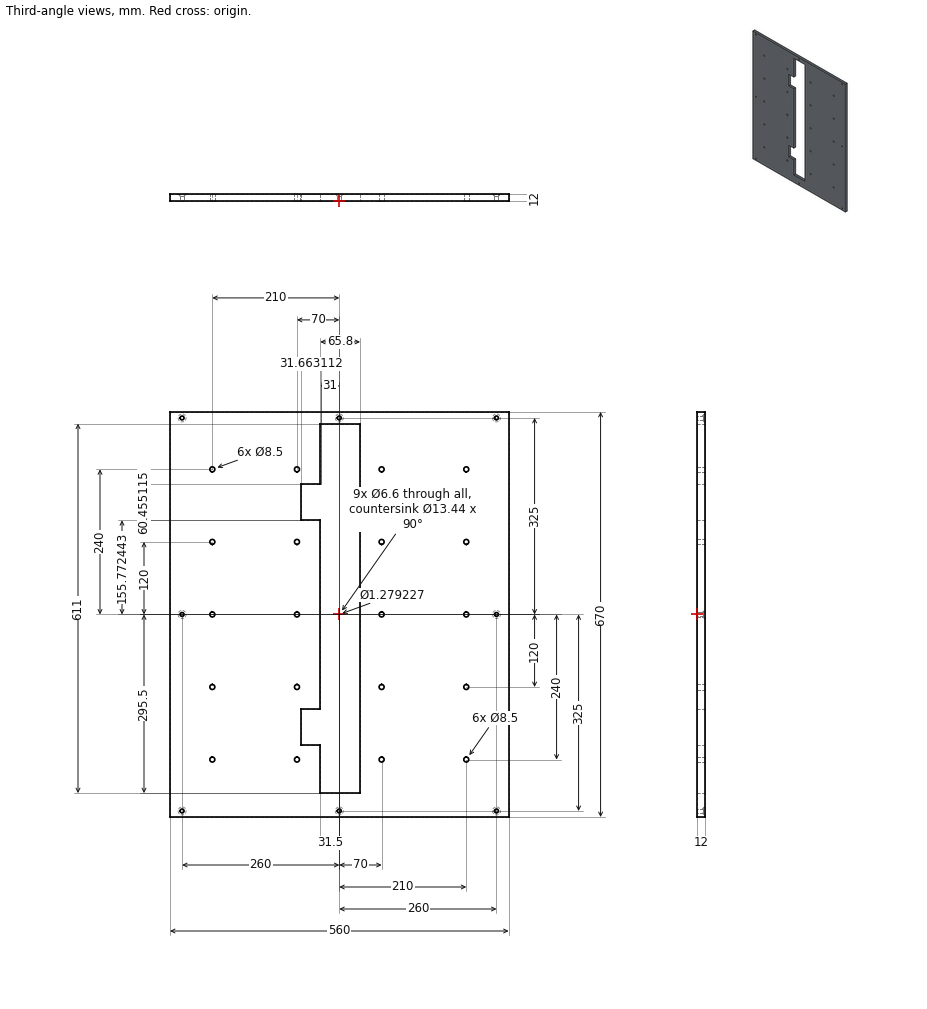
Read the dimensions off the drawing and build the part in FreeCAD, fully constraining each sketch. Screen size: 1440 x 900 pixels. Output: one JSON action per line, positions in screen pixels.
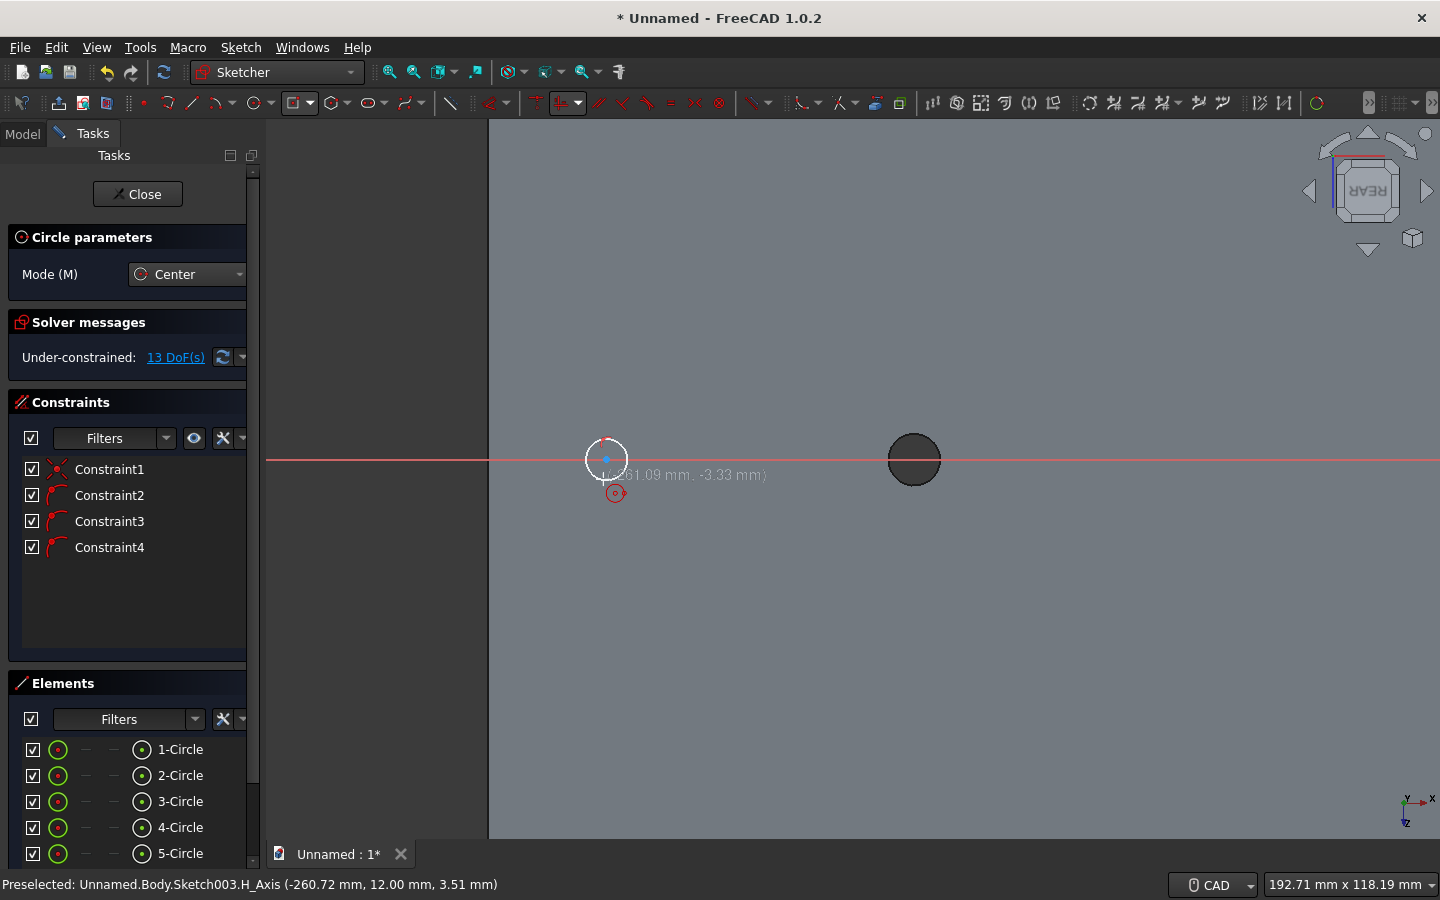
{"action": "scroll", "coordinate": [609, 481], "scroll_direction": "down", "scroll_amount": 11}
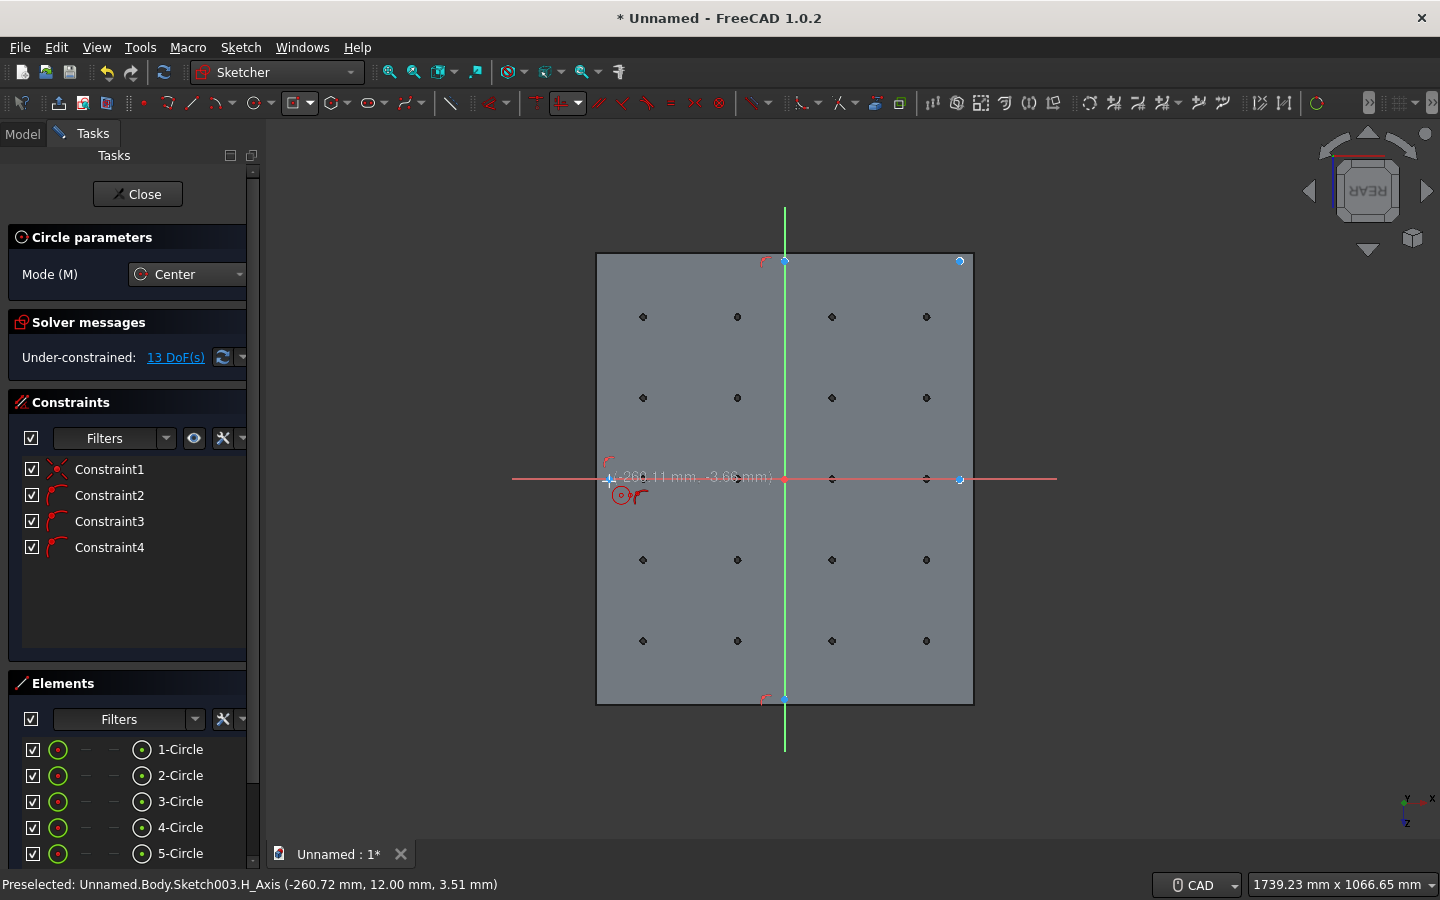
{"action": "scroll", "coordinate": [609, 260], "scroll_direction": "up", "scroll_amount": 12}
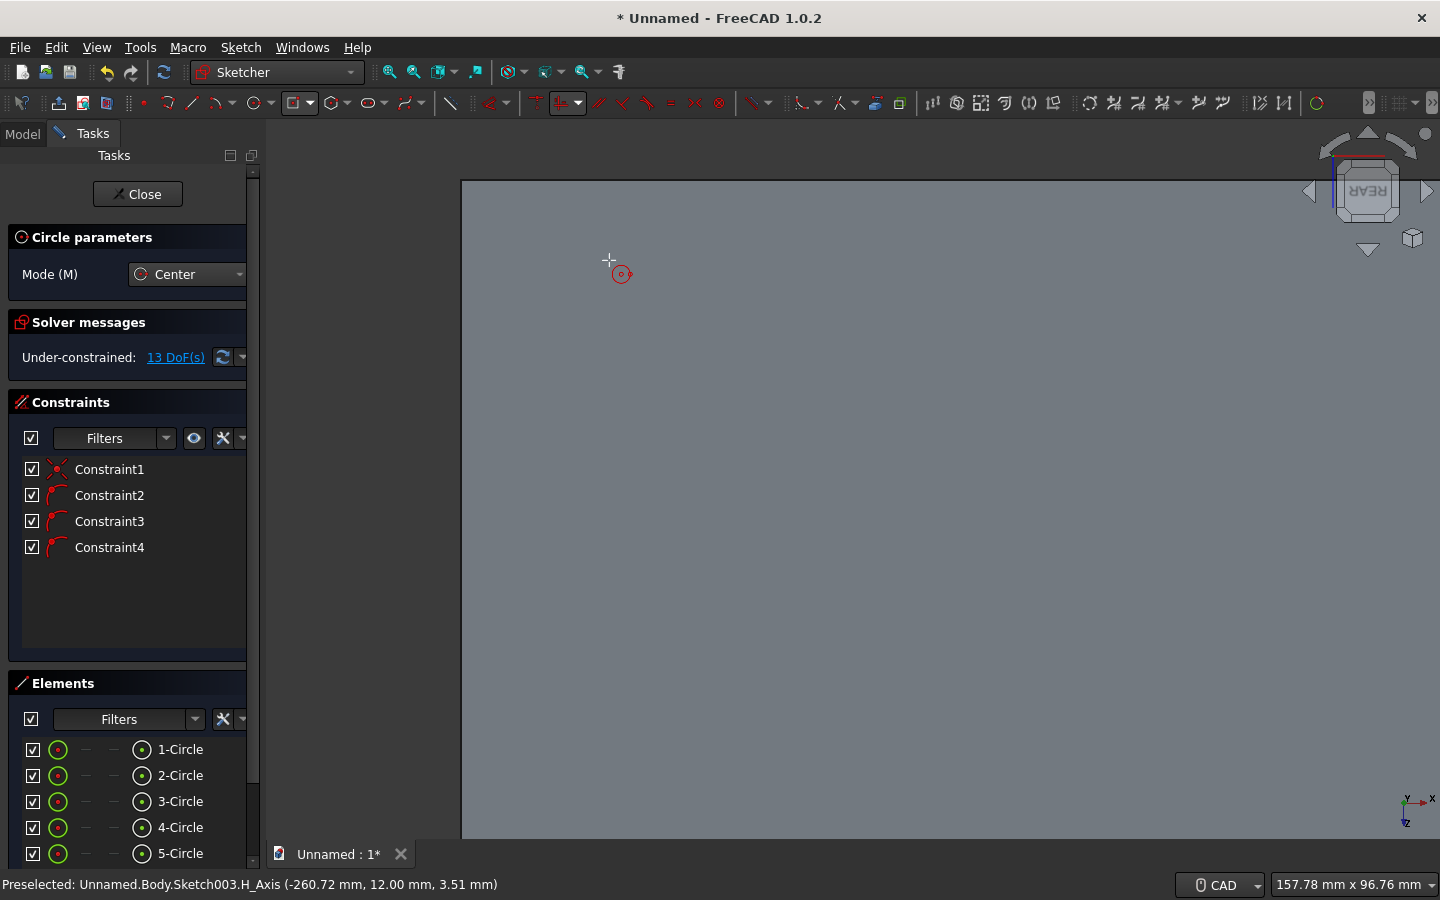
{"action": "scroll", "coordinate": [609, 260], "scroll_direction": "down", "scroll_amount": 12}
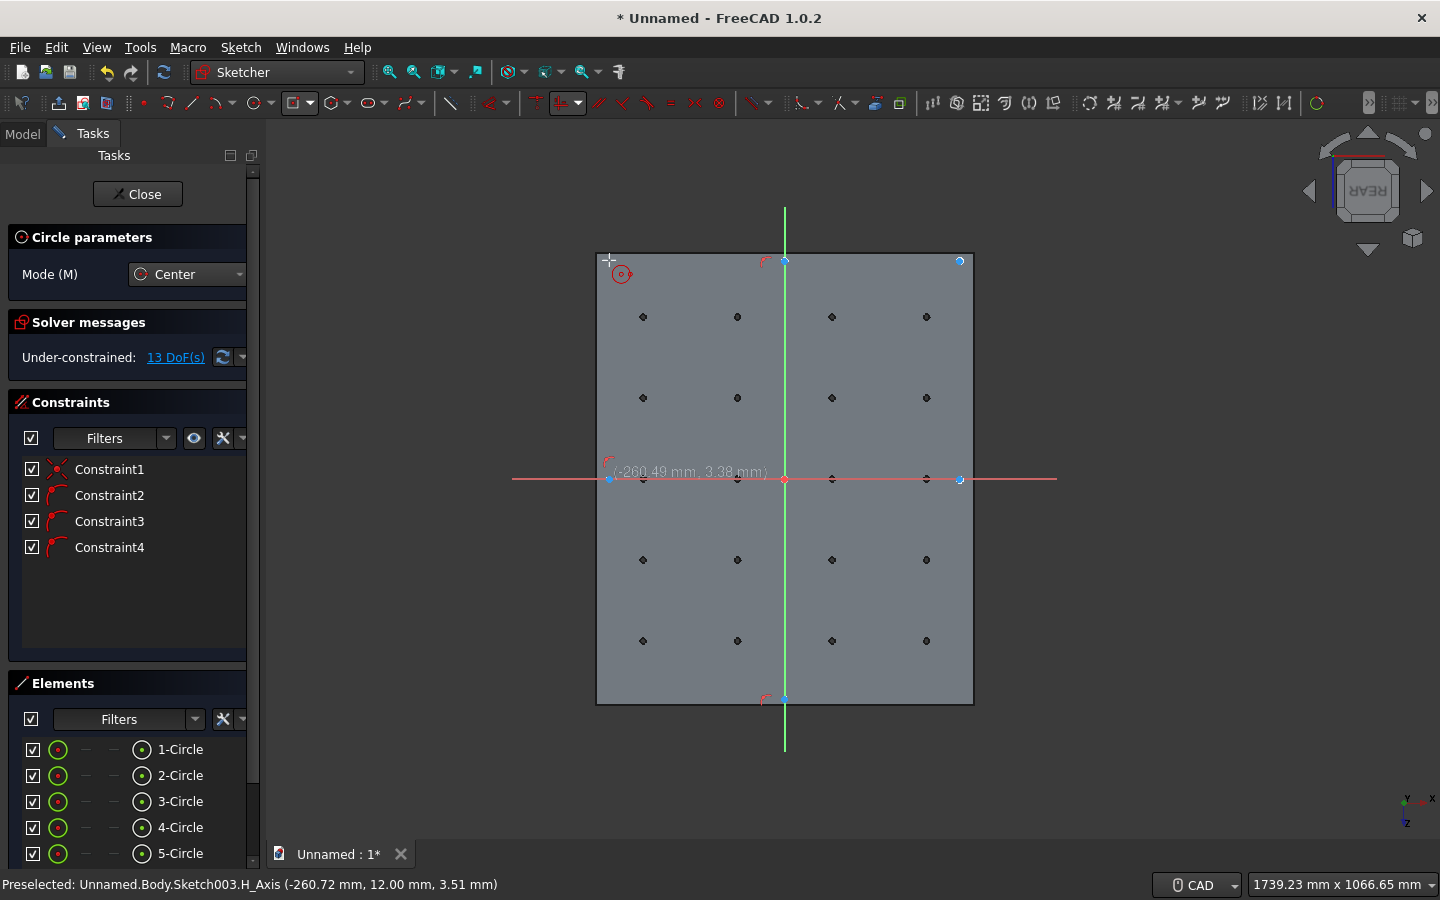
{"action": "left_click", "coordinate": [609, 260]}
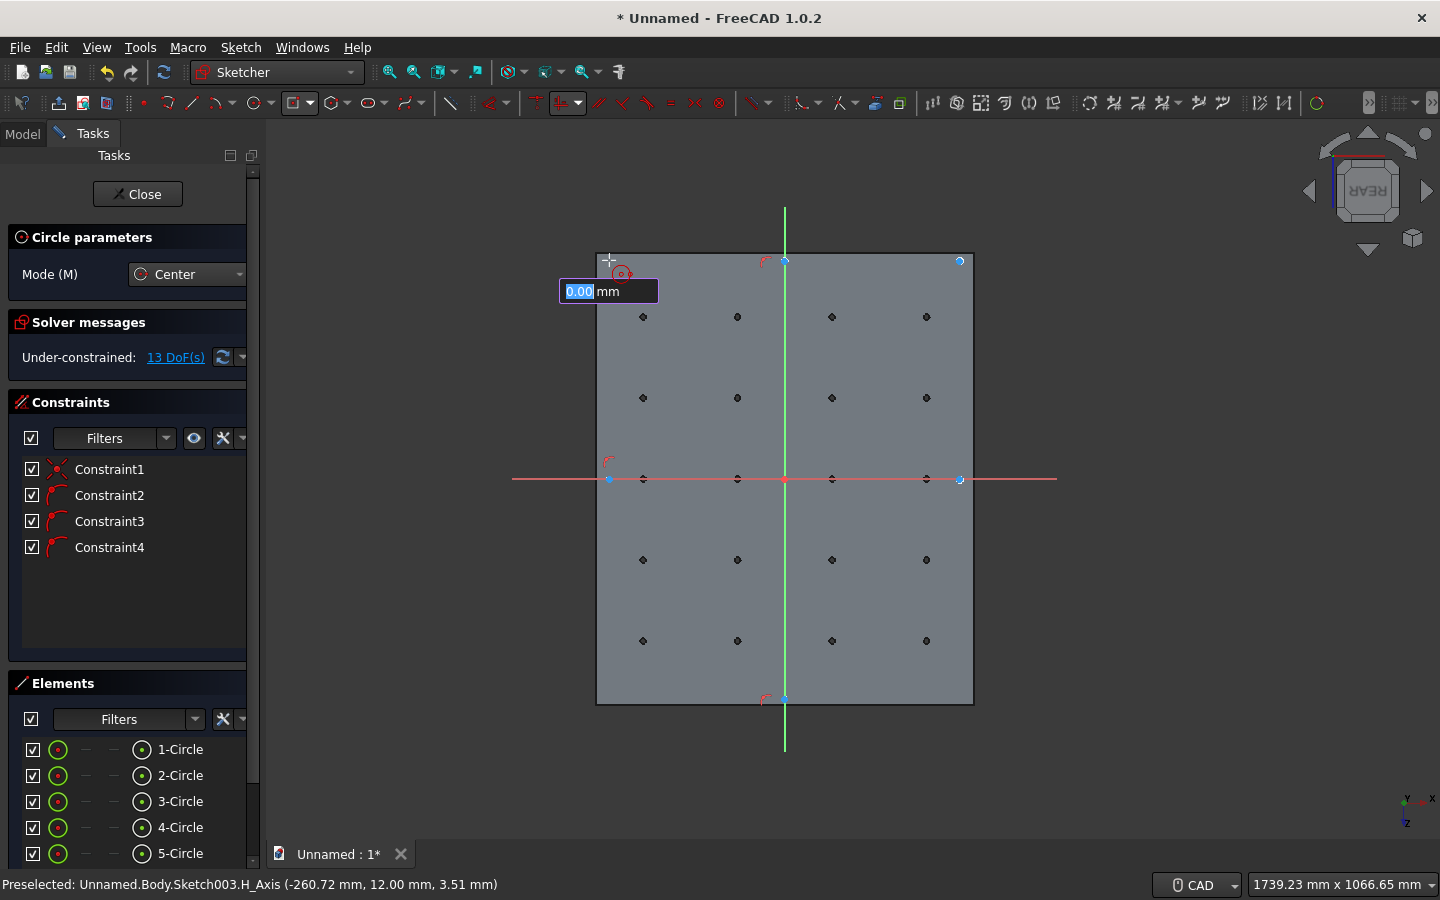
{"action": "scroll", "coordinate": [611, 258], "scroll_direction": "up", "scroll_amount": 10}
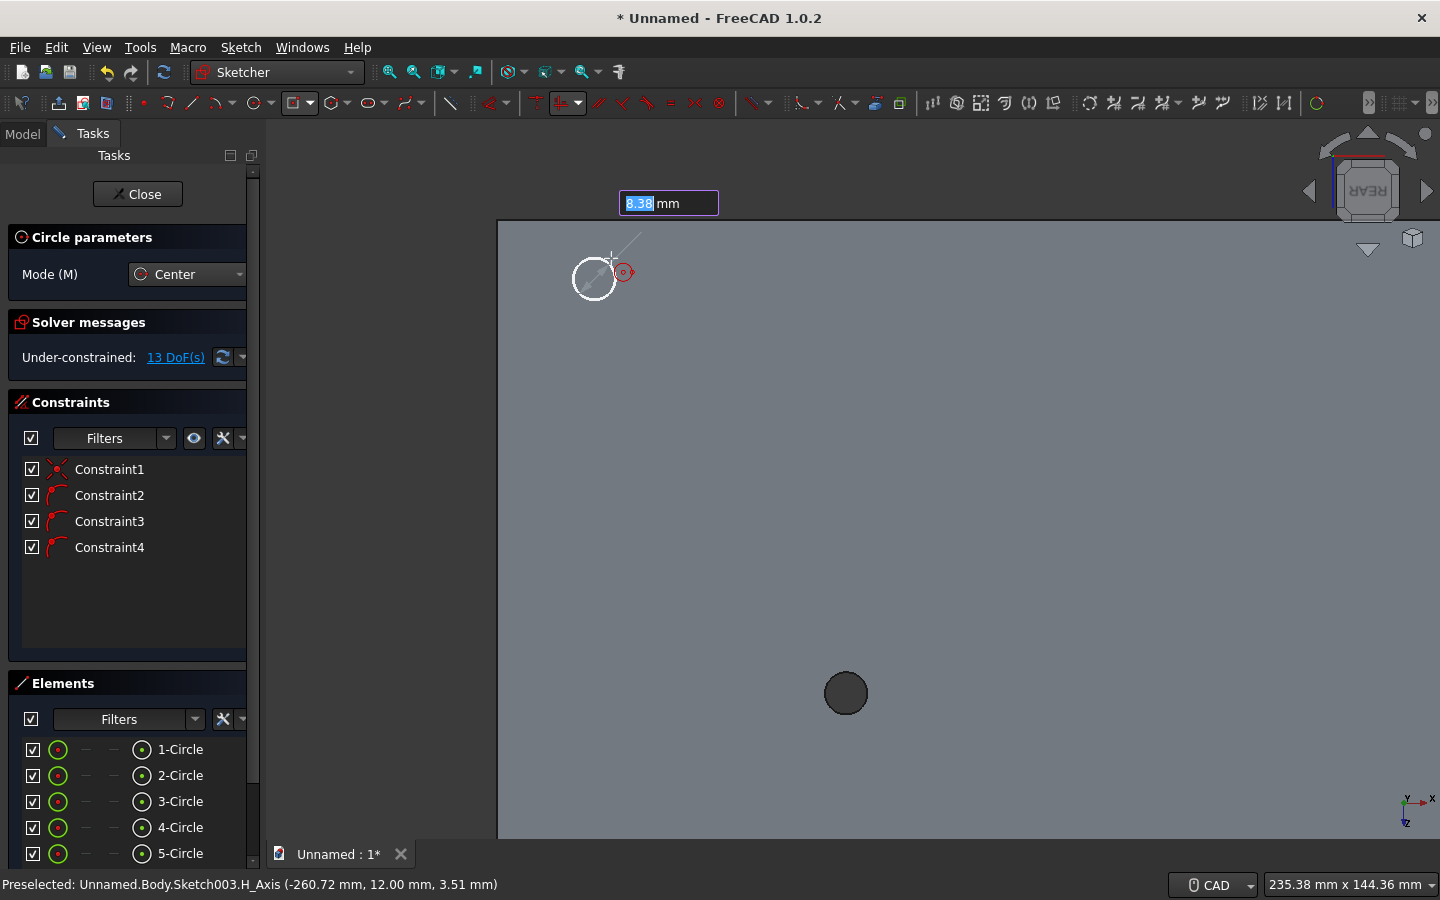
{"action": "left_click", "coordinate": [608, 258]}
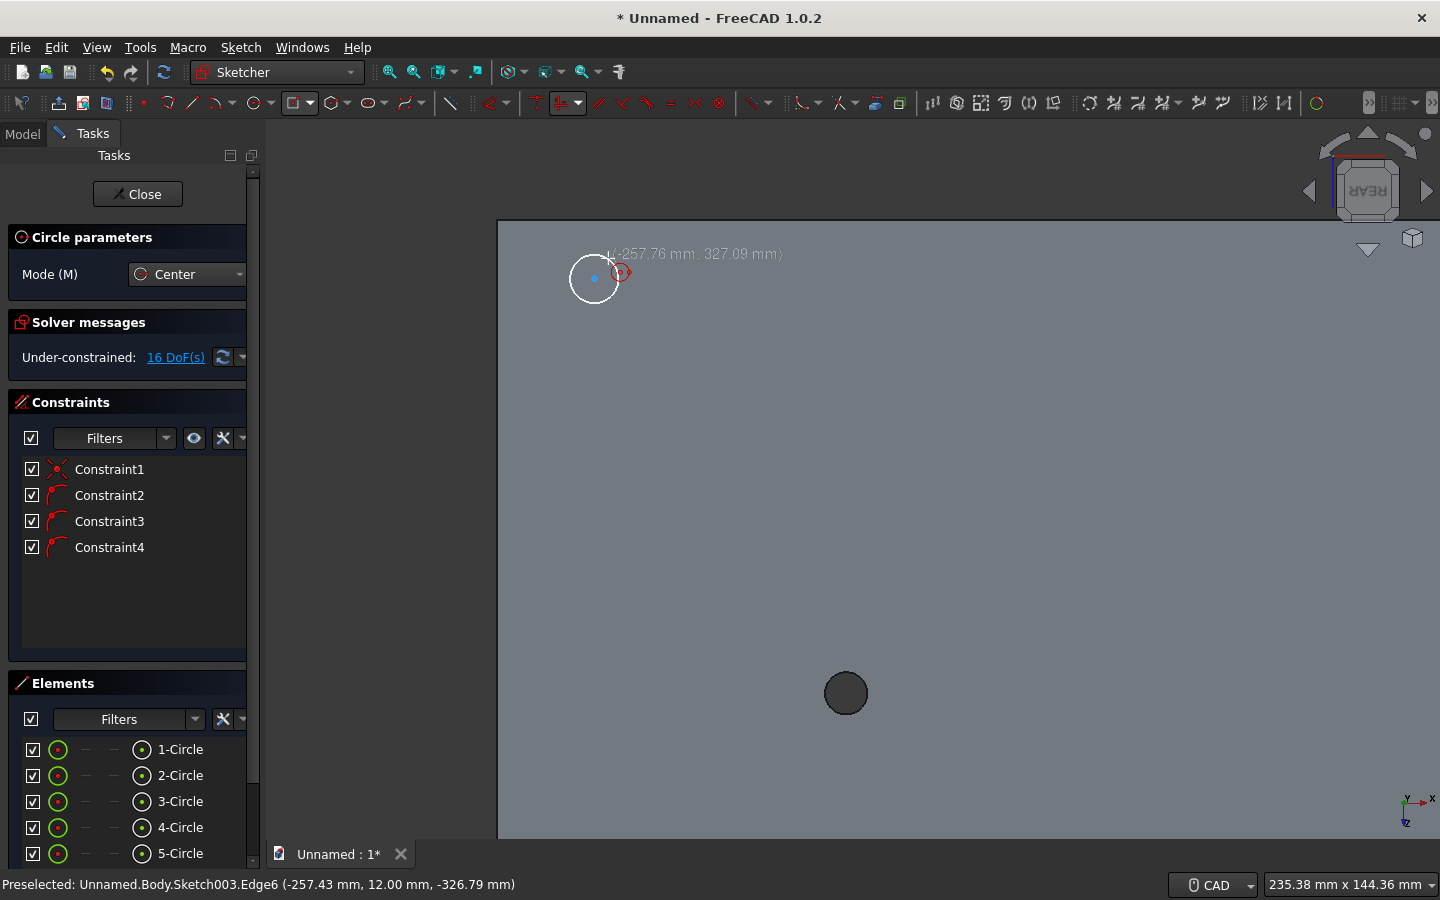
{"action": "scroll", "coordinate": [611, 258], "scroll_direction": "down", "scroll_amount": 10}